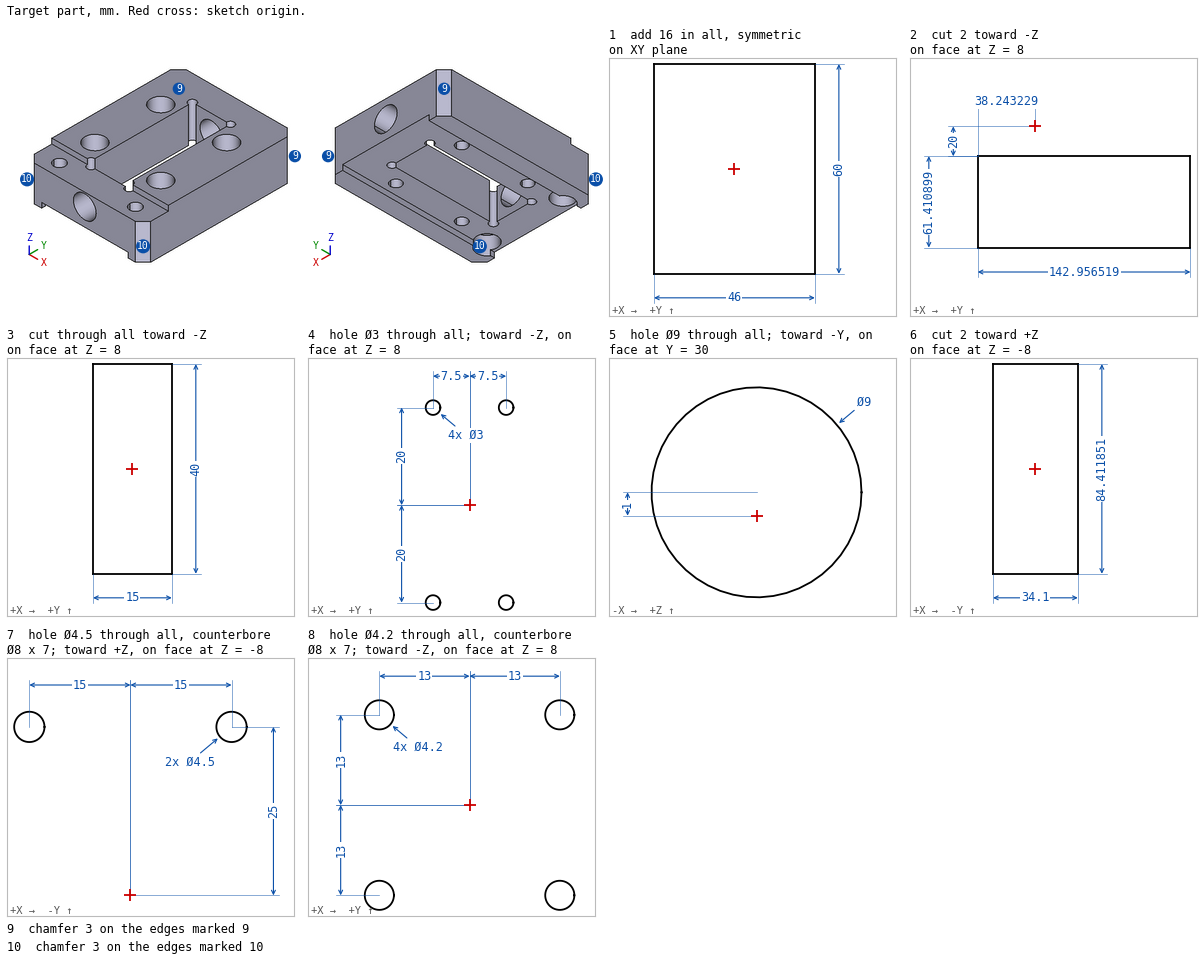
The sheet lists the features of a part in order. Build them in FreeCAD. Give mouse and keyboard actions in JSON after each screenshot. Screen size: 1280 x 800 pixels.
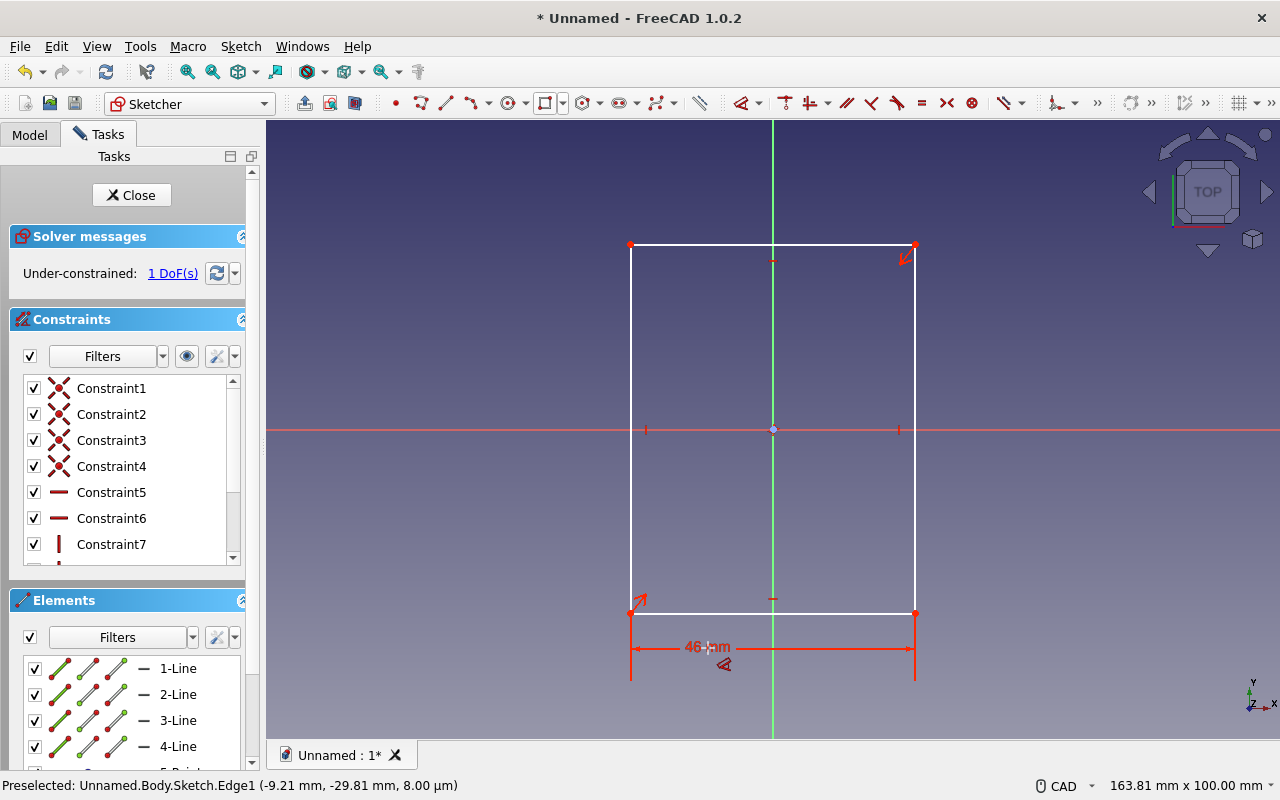
{"action": "left_click", "coordinate": [915, 503]}
{"action": "left_click", "coordinate": [949, 345]}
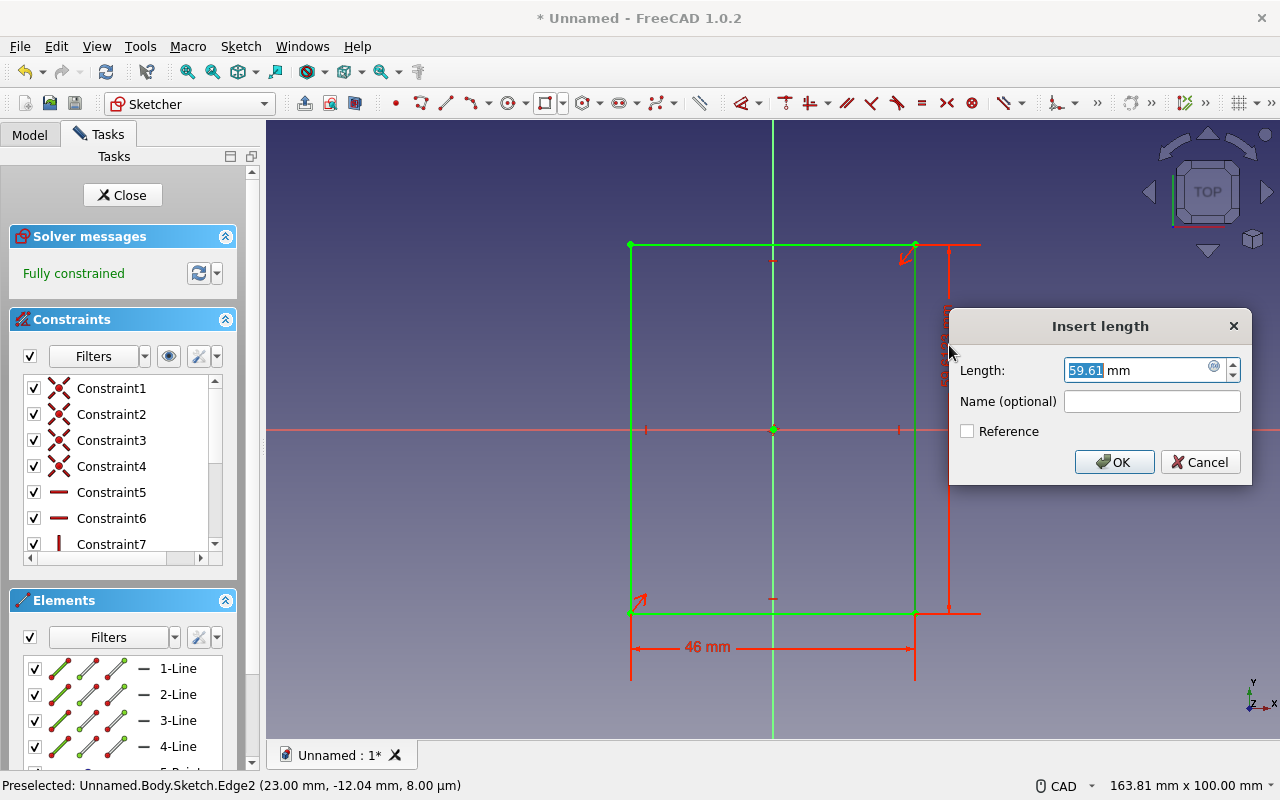
{"action": "type", "text": "60"}
{"action": "key", "text": "Return"}
{"action": "key", "text": "Escape"}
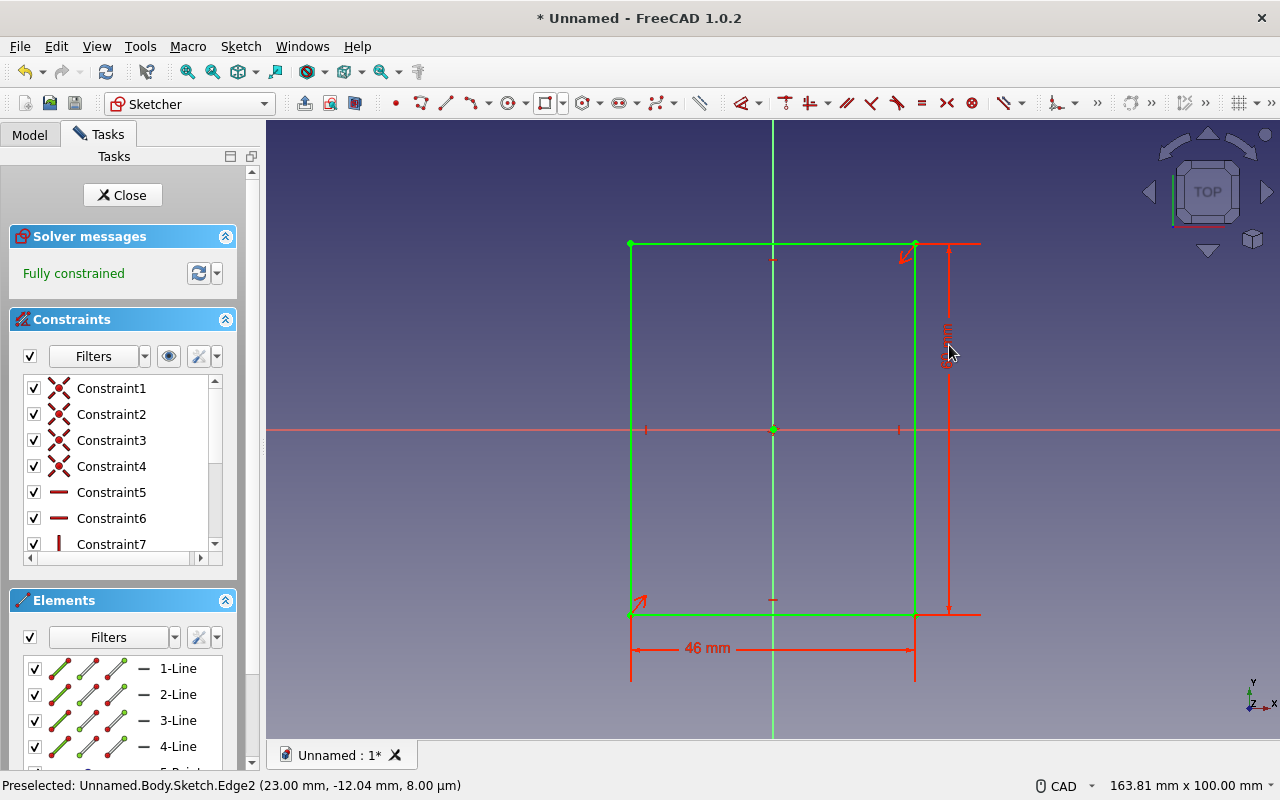
{"action": "left_click", "coordinate": [123, 195]}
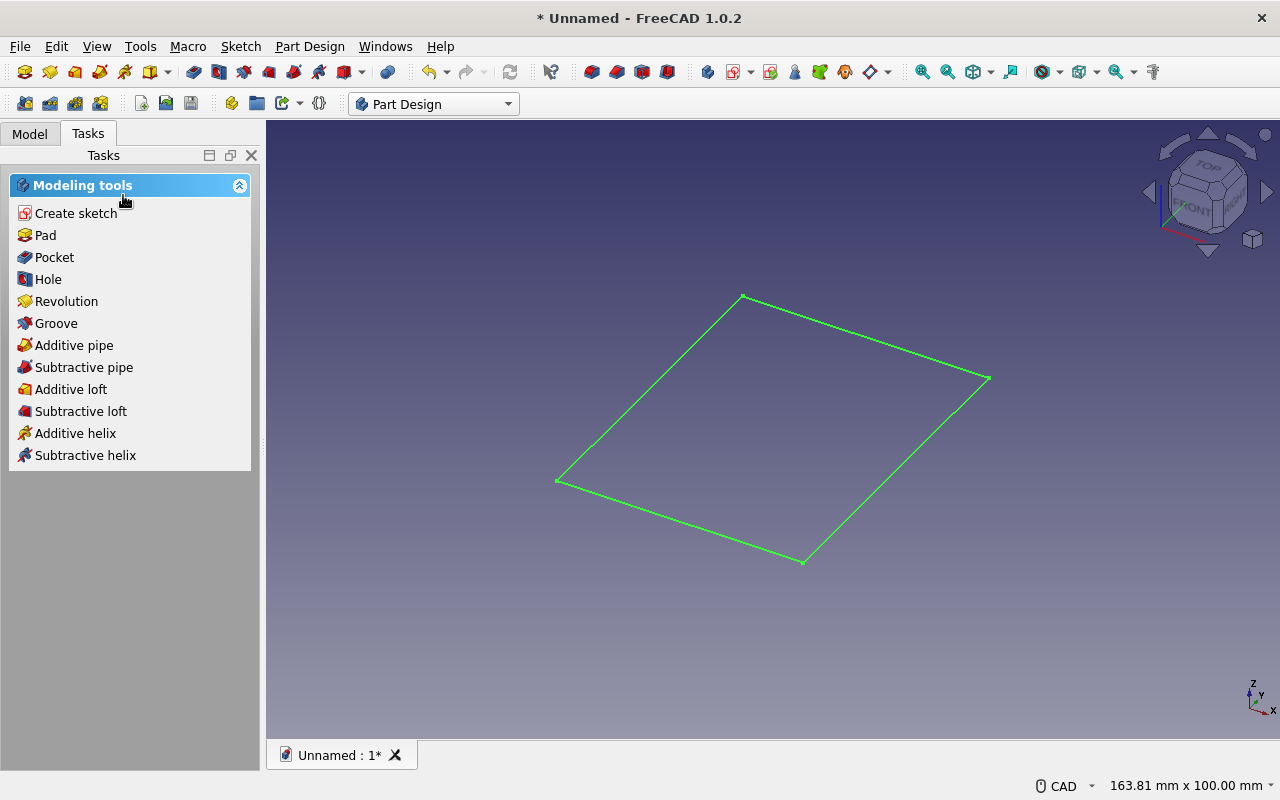
{"action": "left_click", "coordinate": [25, 72]}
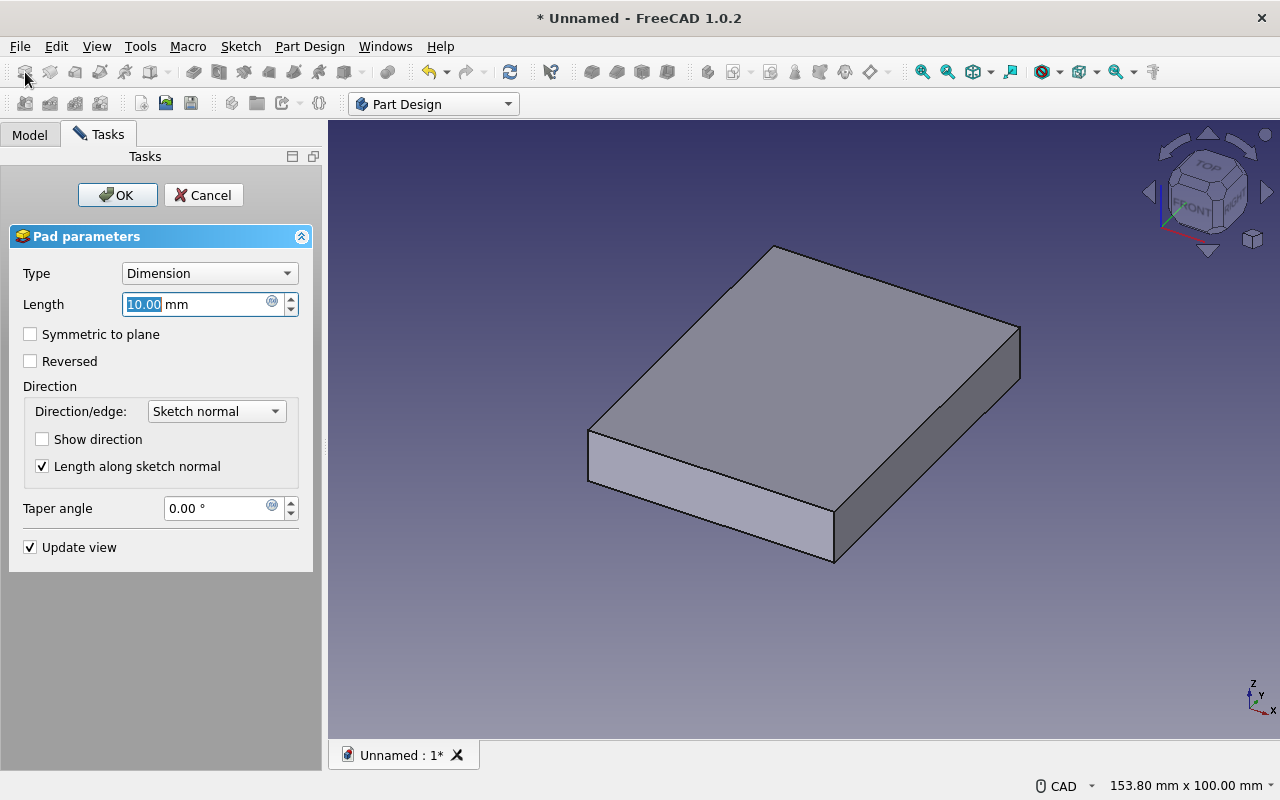
{"action": "type", "text": "16"}
{"action": "key", "text": "Tab"}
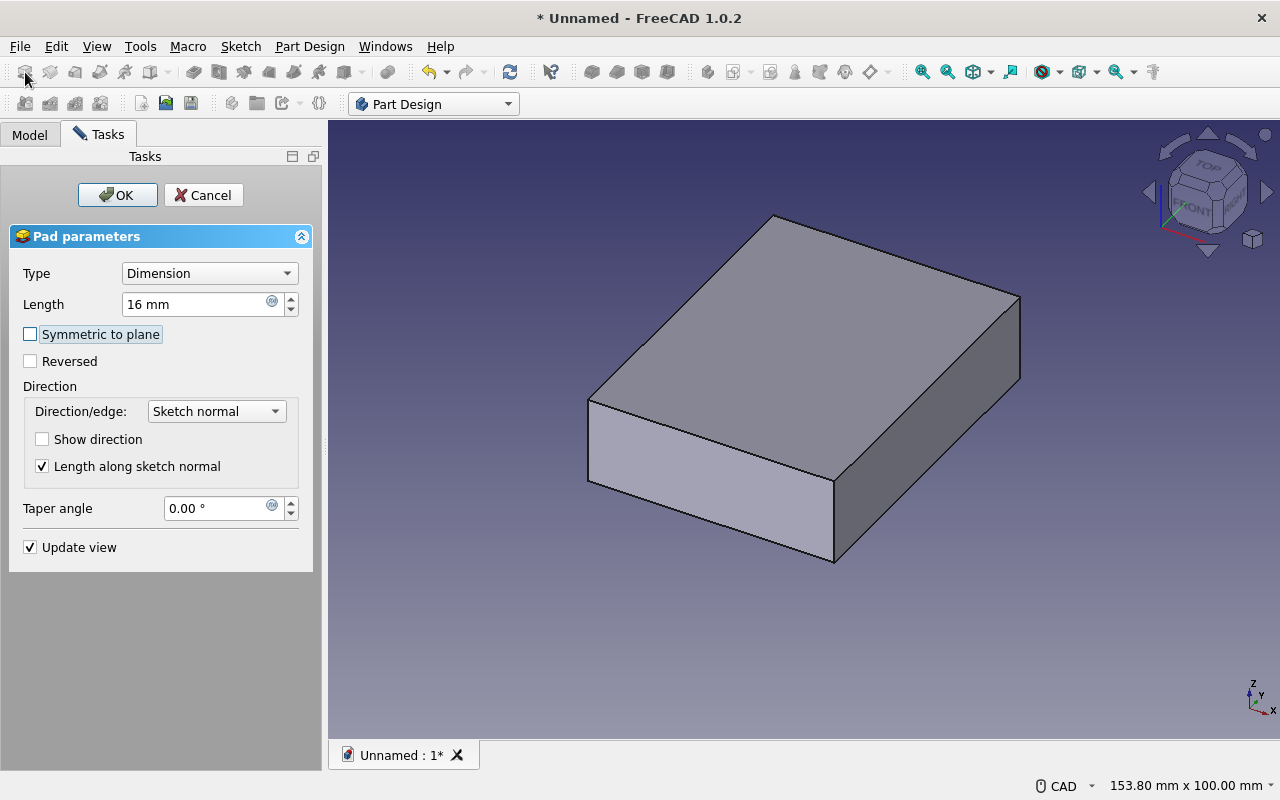
{"action": "left_click", "coordinate": [31, 334]}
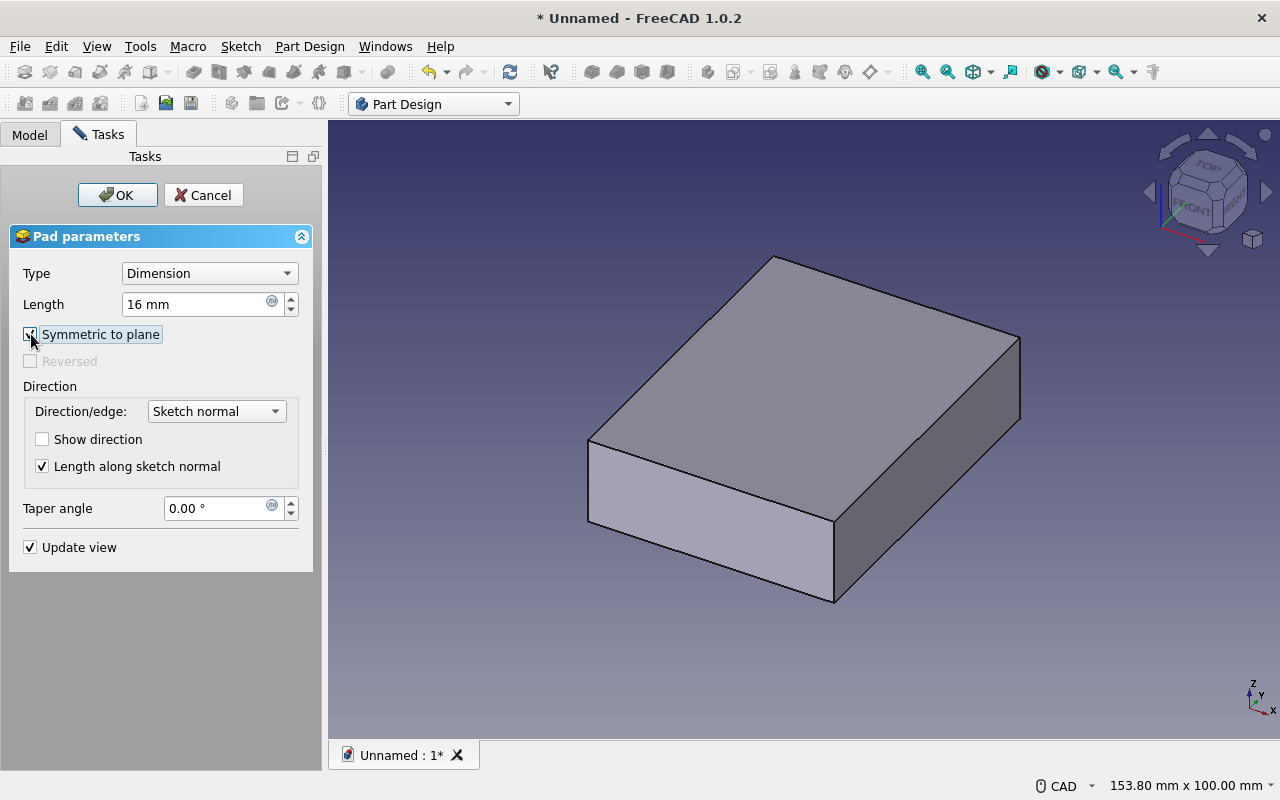
{"action": "left_click", "coordinate": [118, 195]}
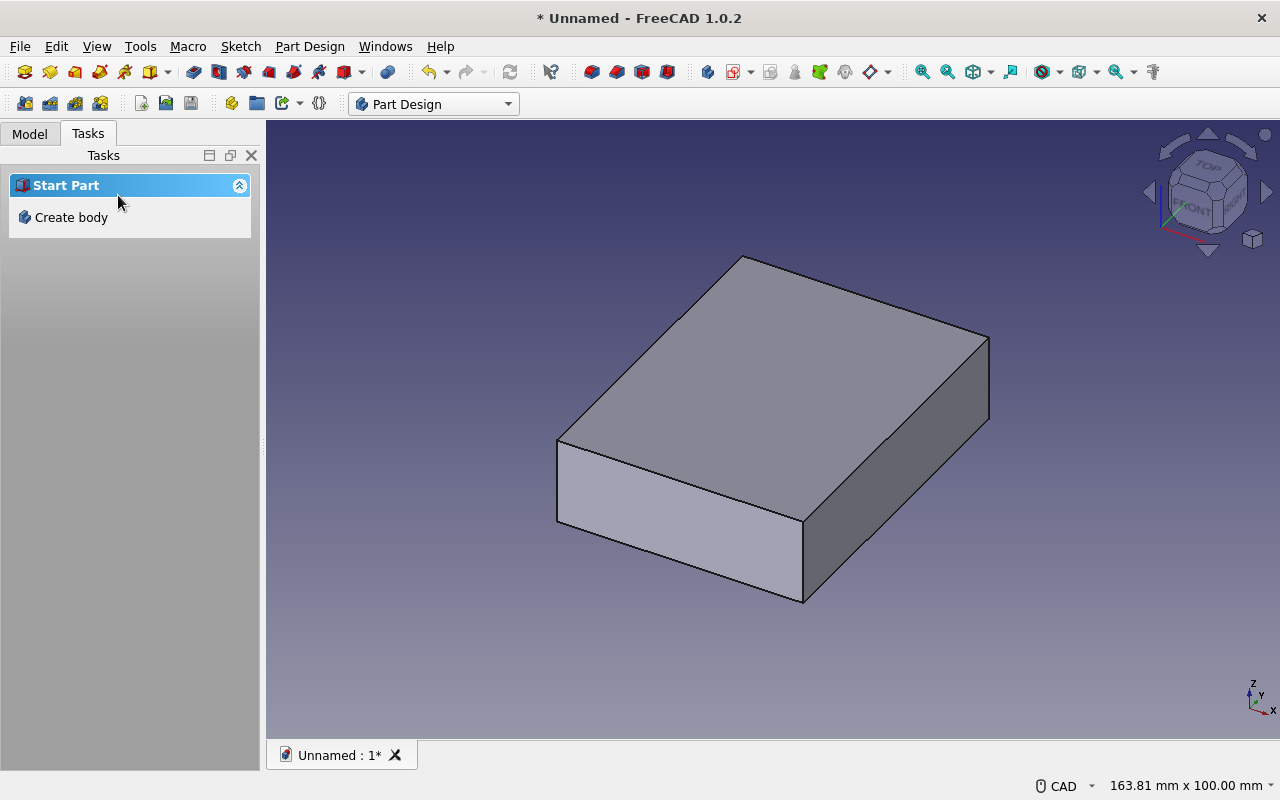
{"action": "left_click", "coordinate": [773, 388]}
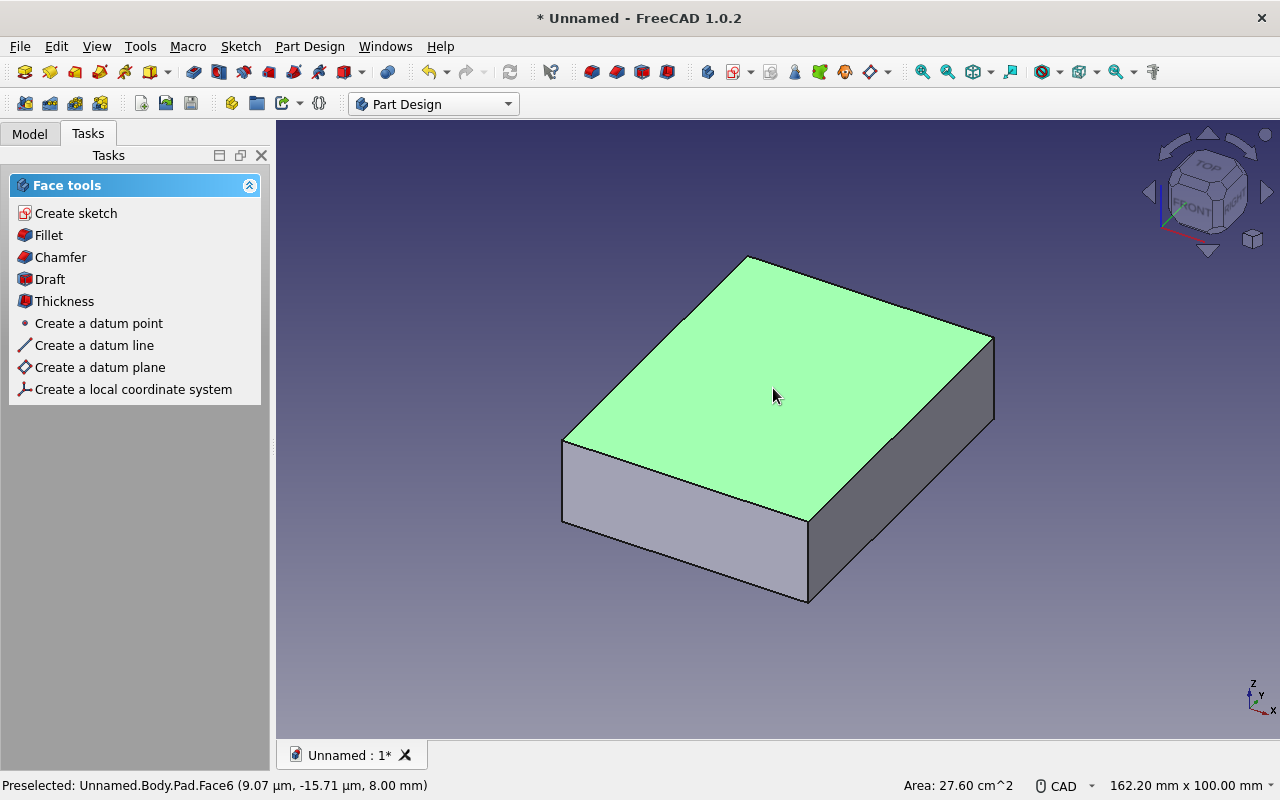
{"action": "left_click", "coordinate": [732, 72]}